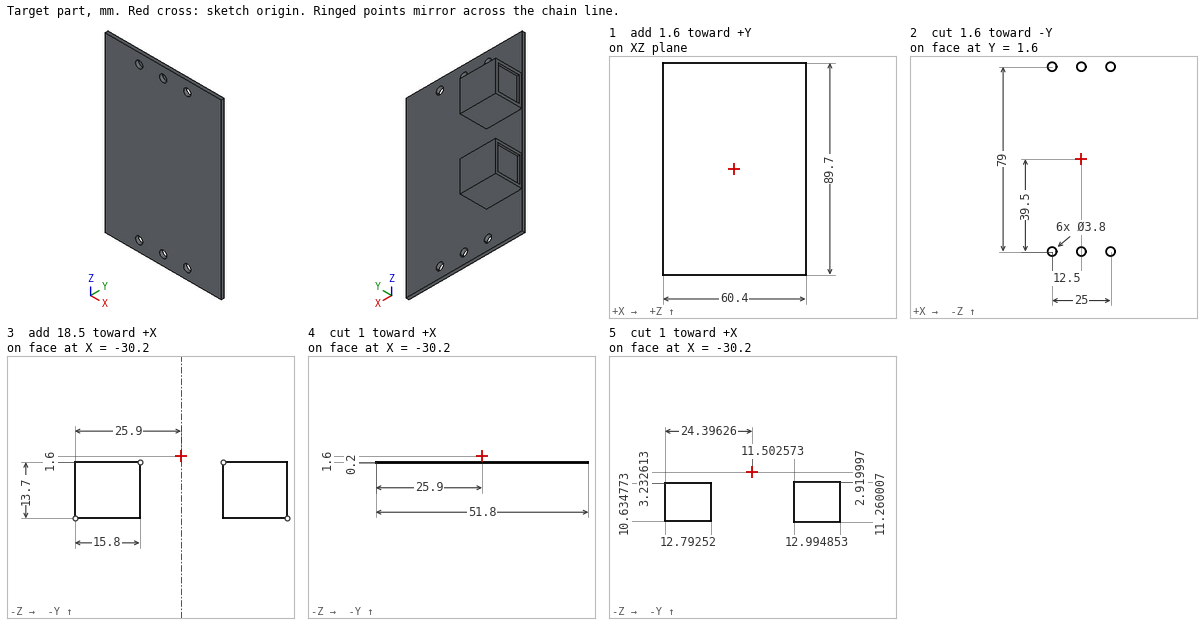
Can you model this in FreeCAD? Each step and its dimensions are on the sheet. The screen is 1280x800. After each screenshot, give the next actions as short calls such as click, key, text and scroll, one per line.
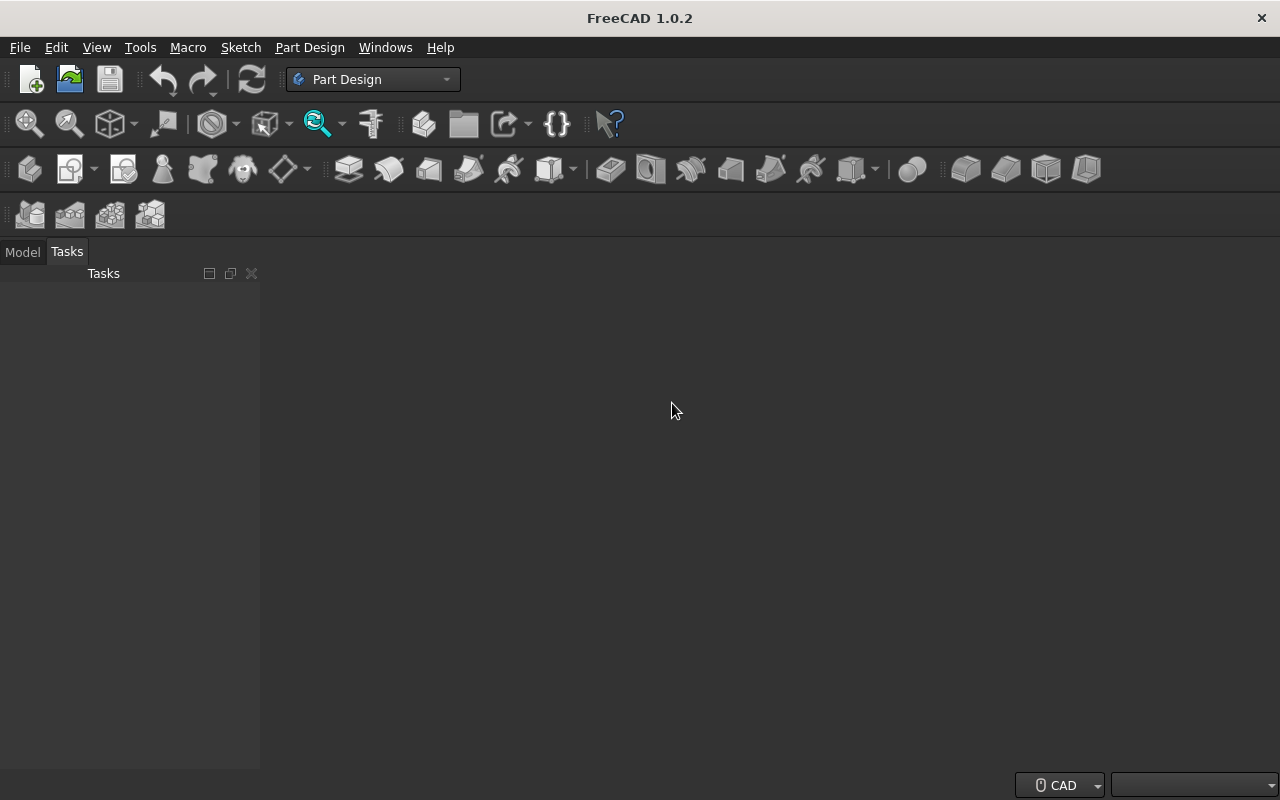
key(ctrl+n)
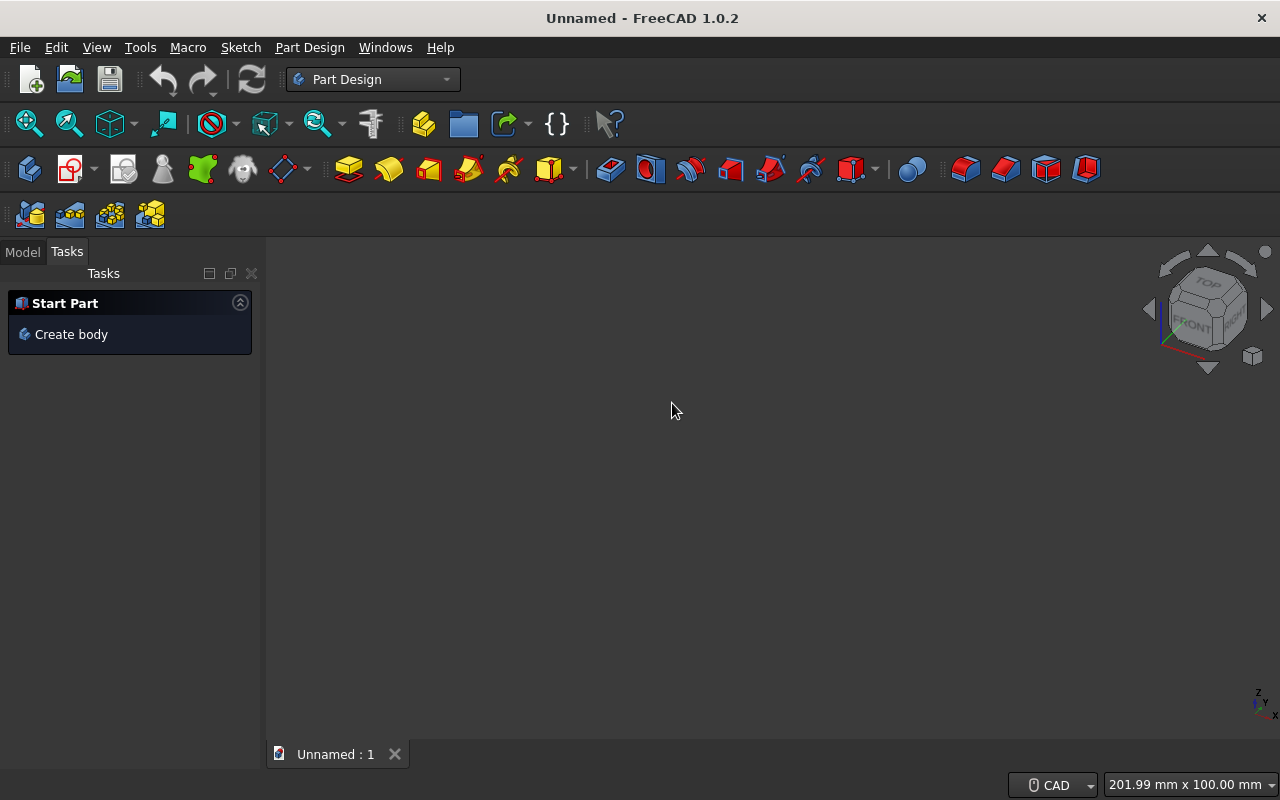
click(70, 170)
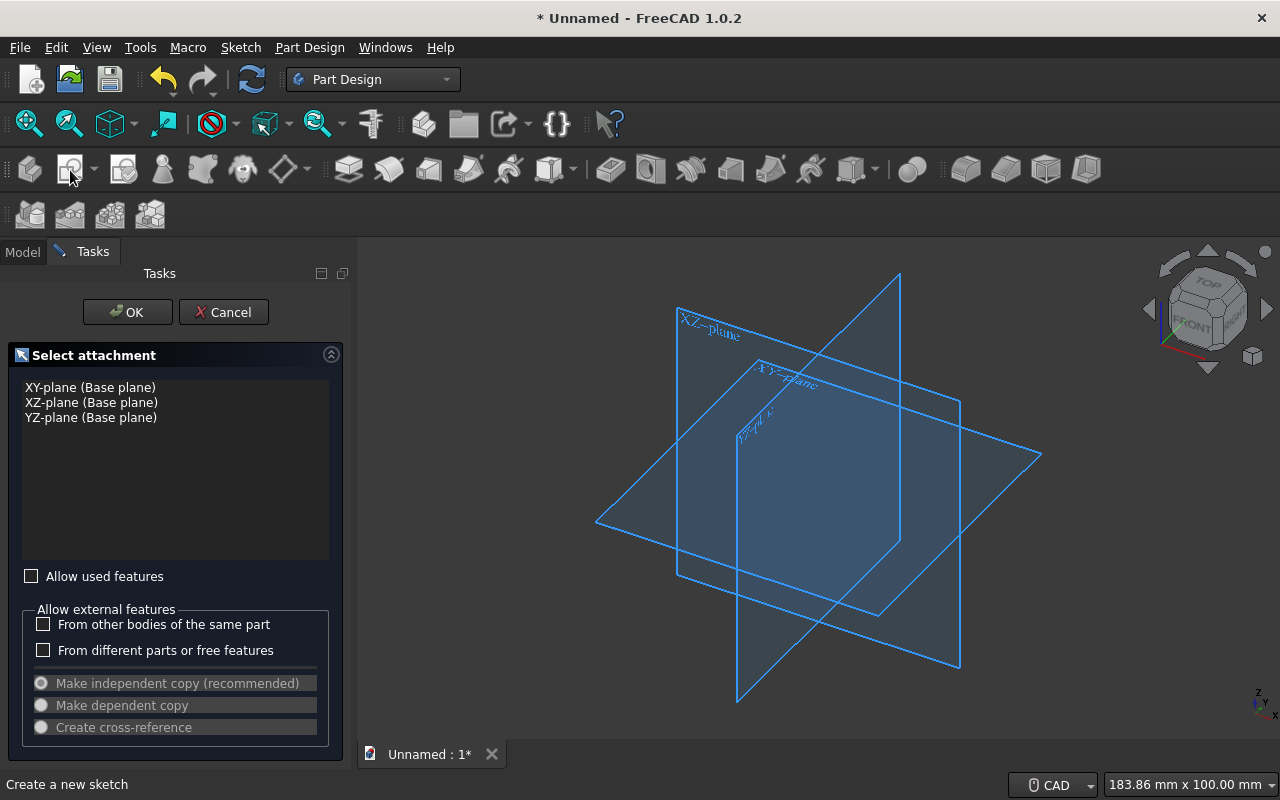
click(82, 402)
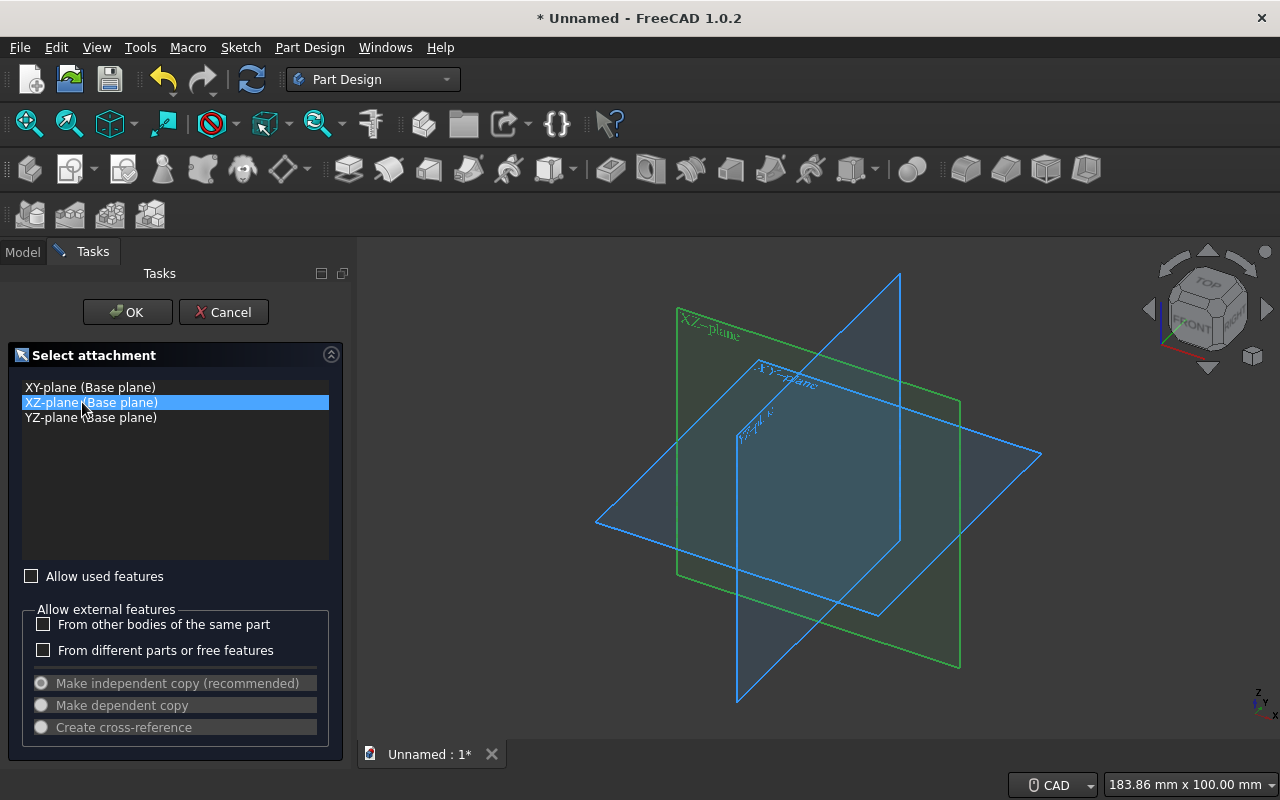
click(128, 312)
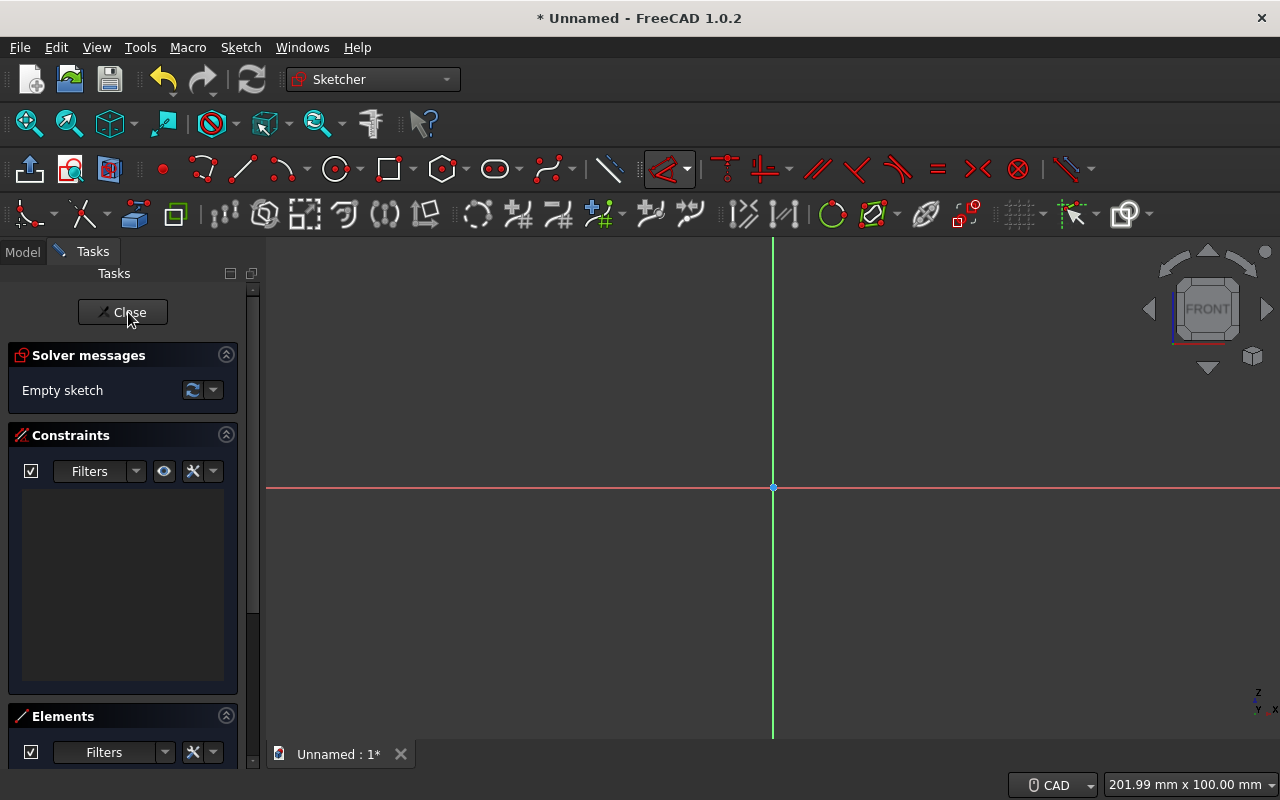
scroll(565, 488, down, 2)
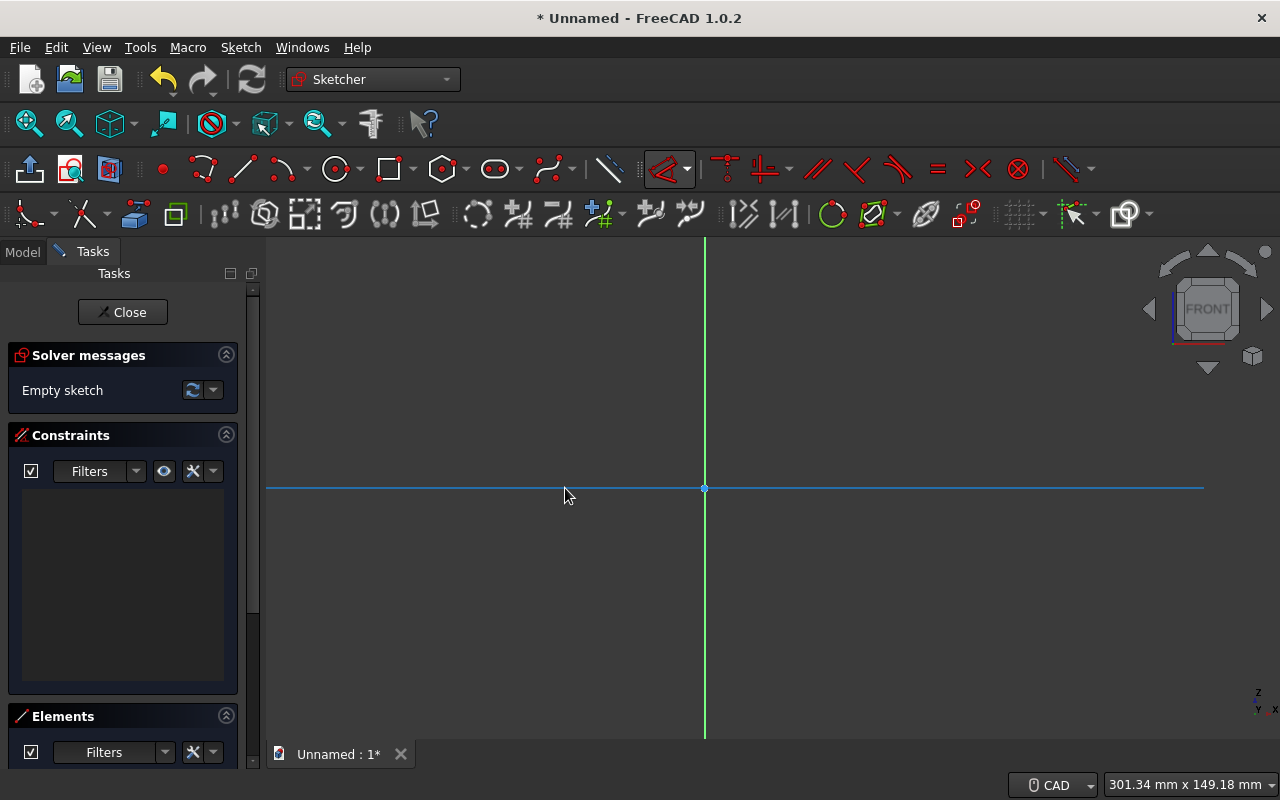
key(g)
key(v)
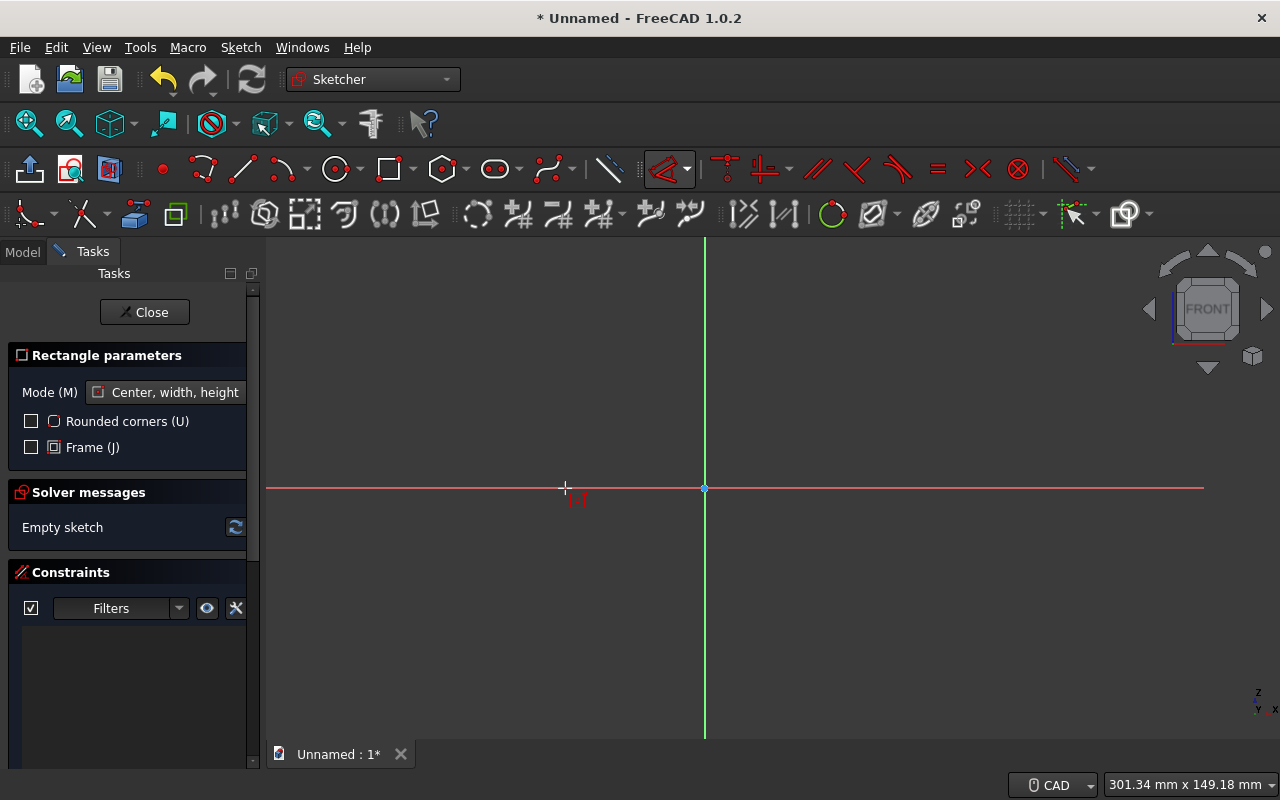
click(705, 488)
click(806, 337)
key(Escape)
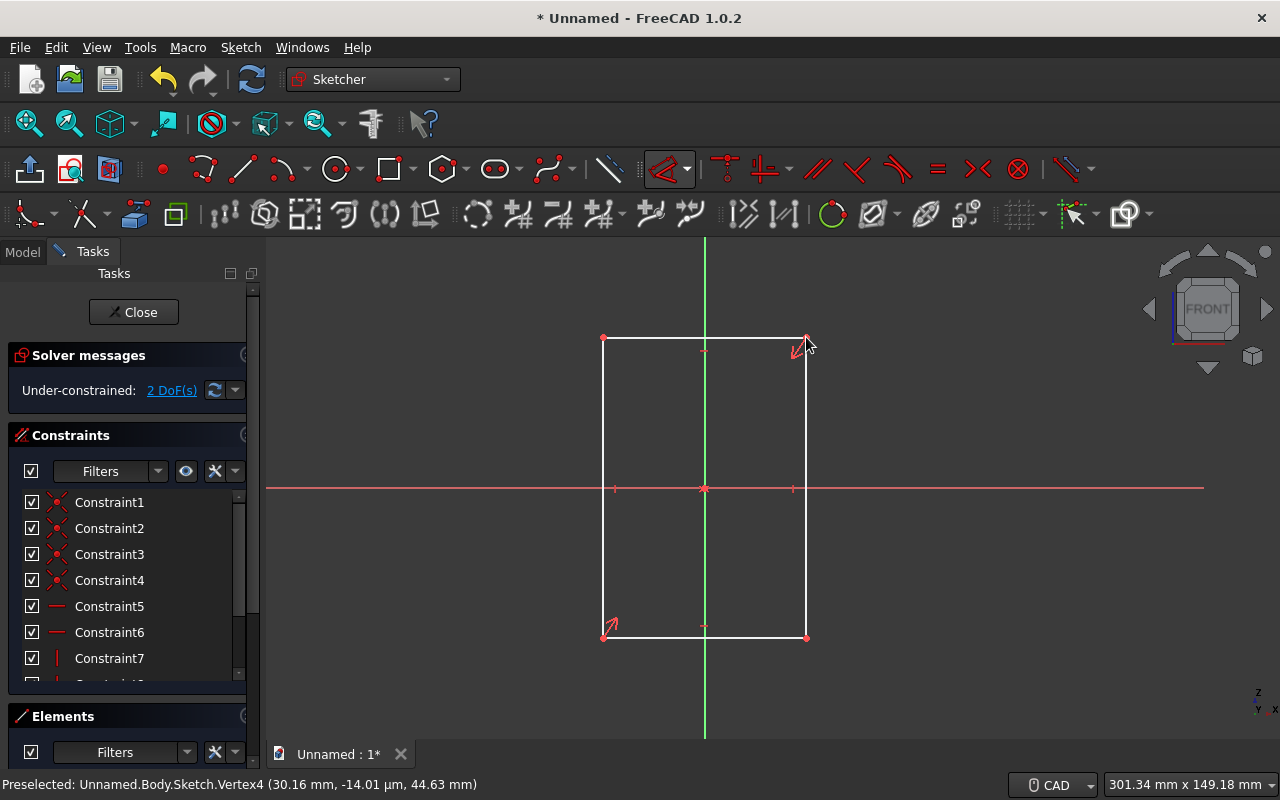
key(d)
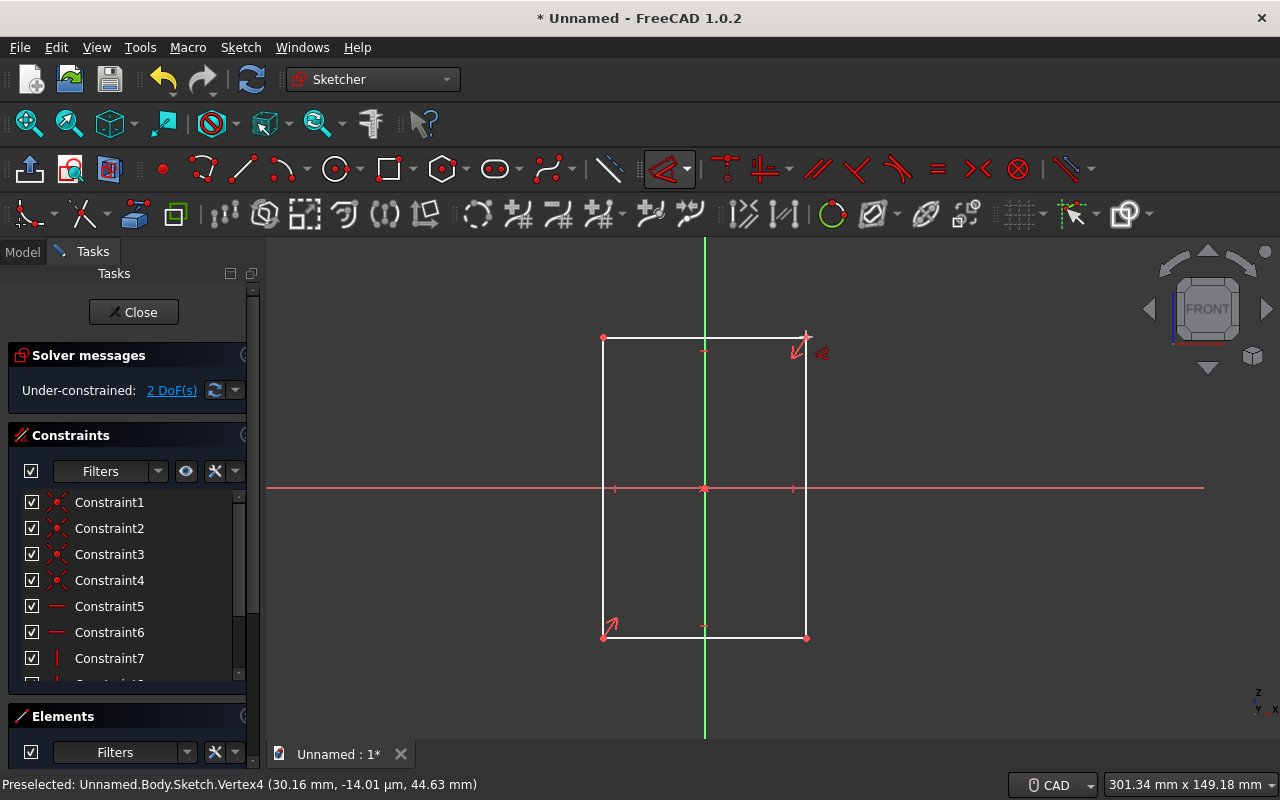
click(664, 638)
click(658, 672)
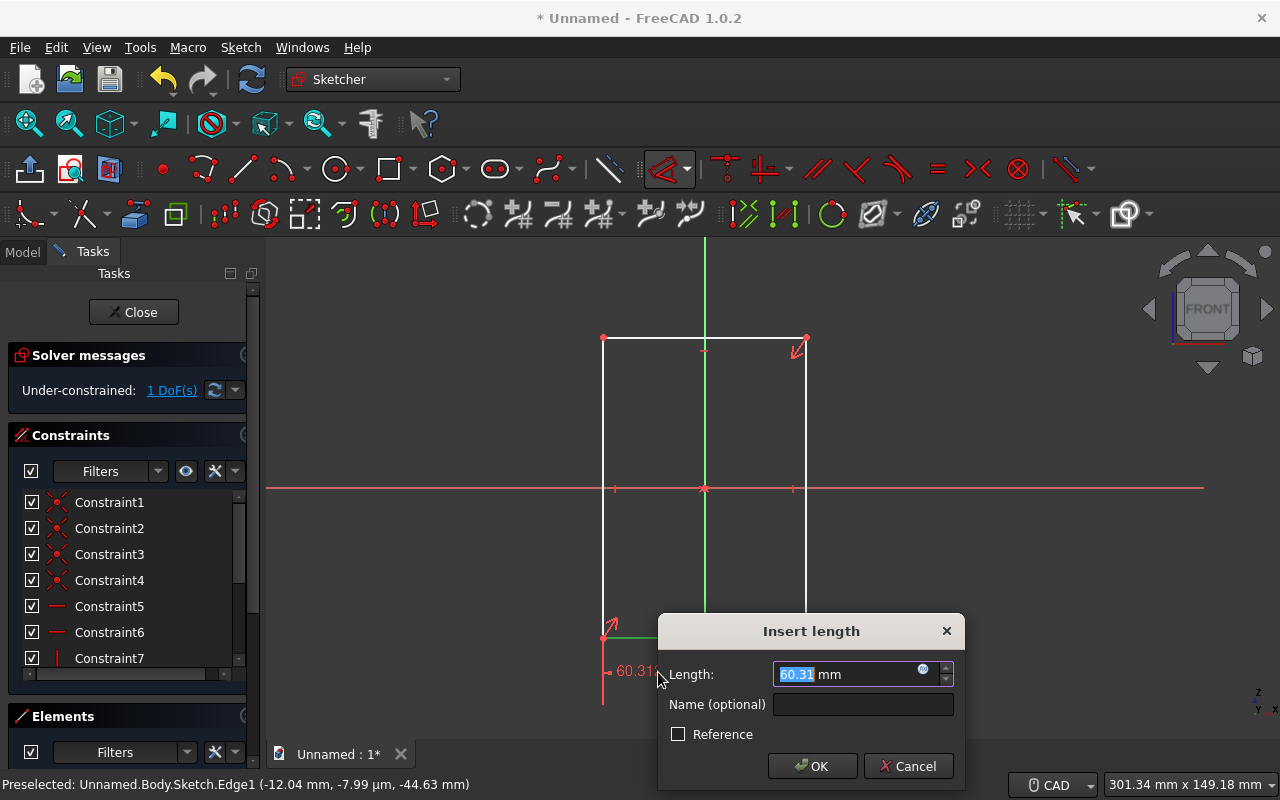
text(60.4)
key(Return)